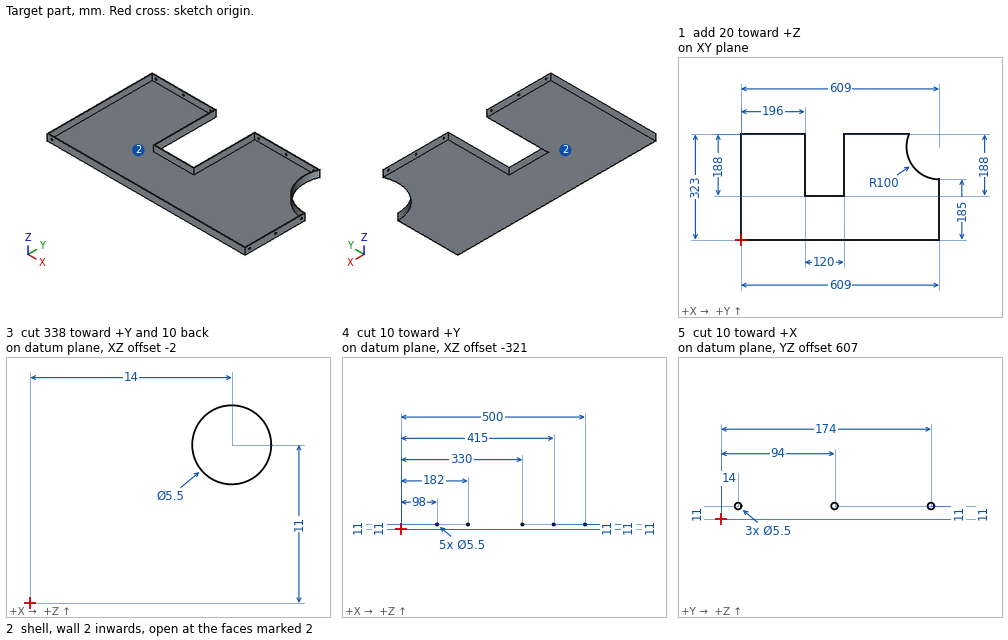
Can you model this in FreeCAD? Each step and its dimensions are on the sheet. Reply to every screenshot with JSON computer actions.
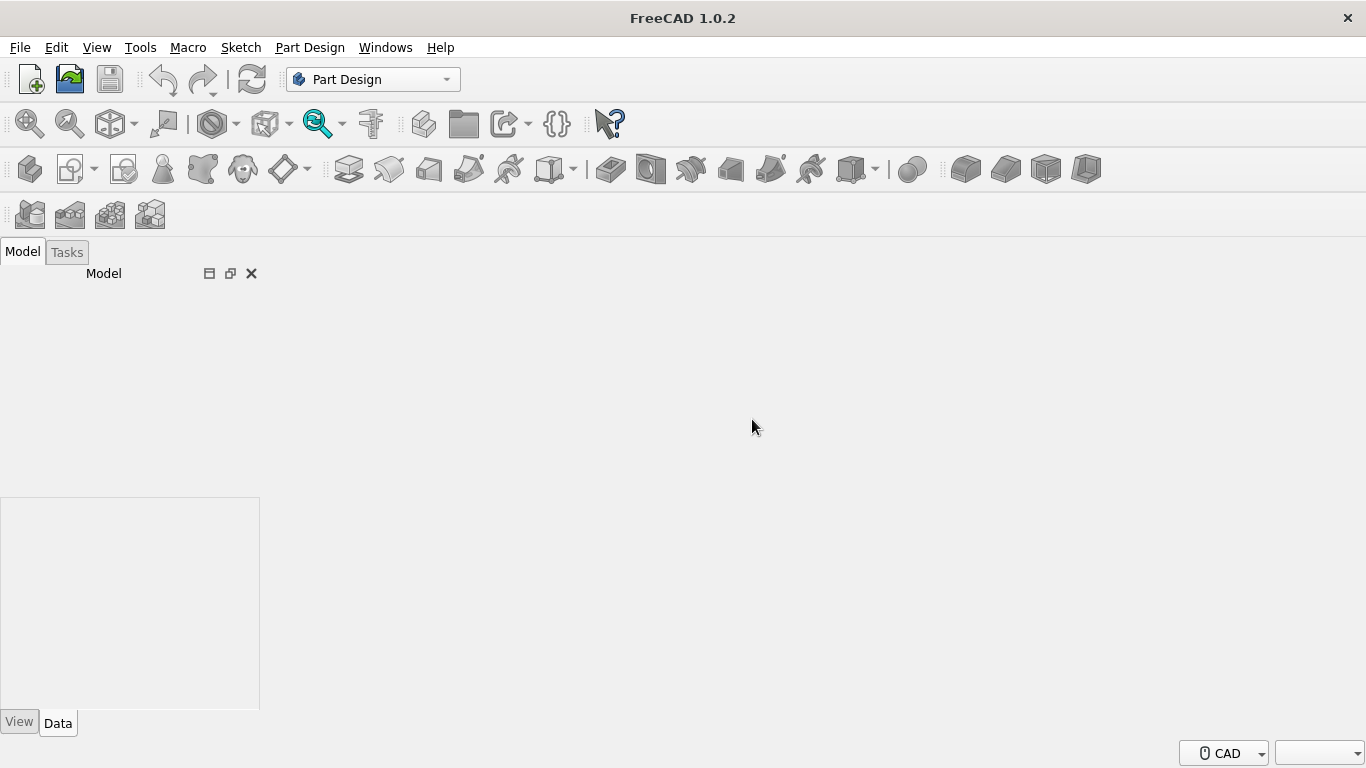
{"action": "key", "text": "ctrl+n"}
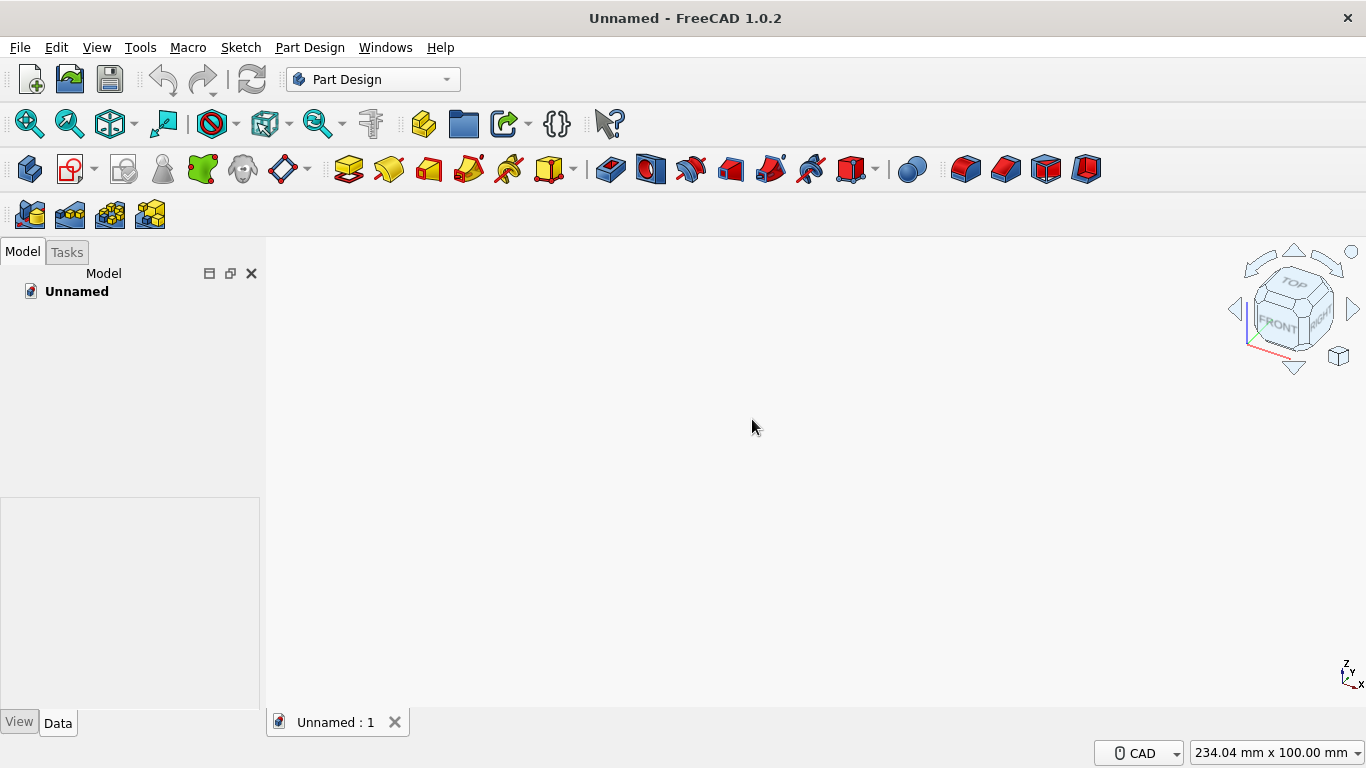
{"action": "left_click", "coordinate": [70, 170]}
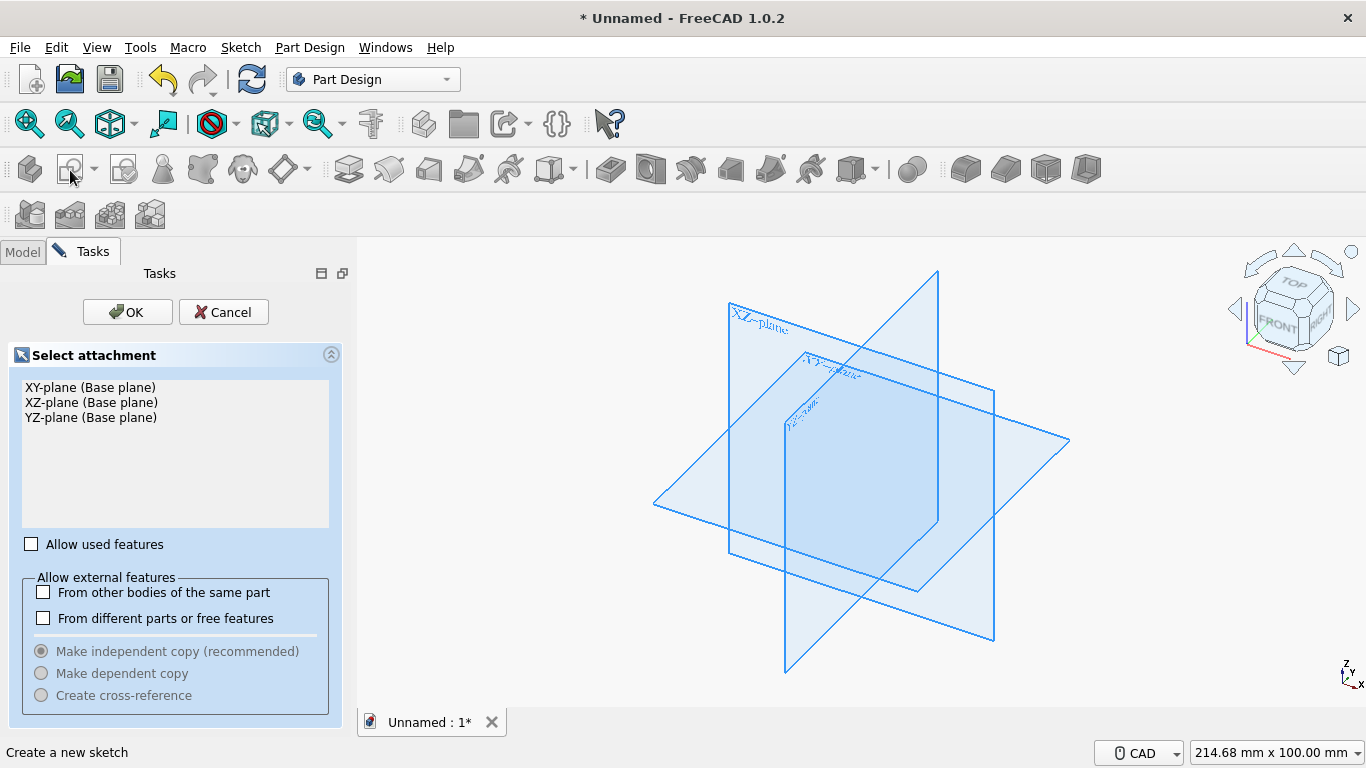
{"action": "left_click", "coordinate": [82, 388]}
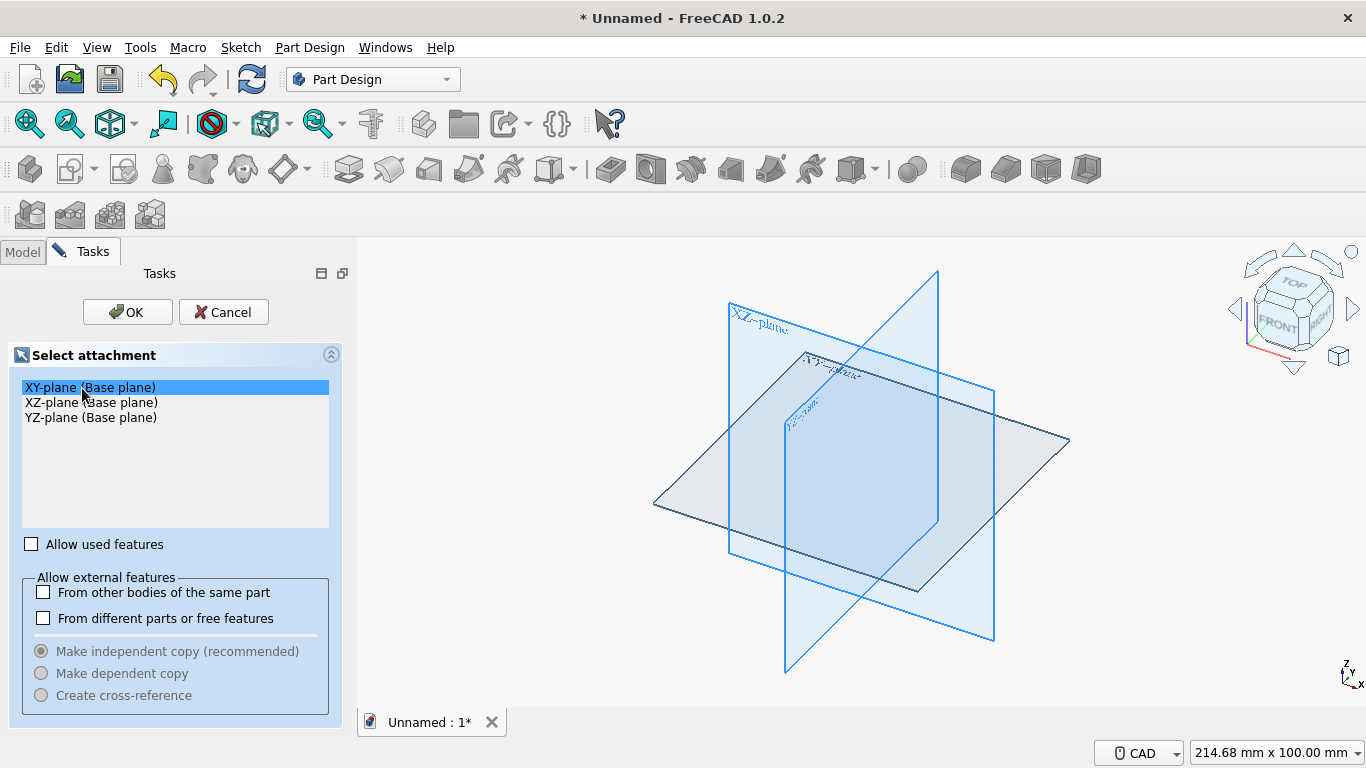
{"action": "left_click", "coordinate": [128, 312]}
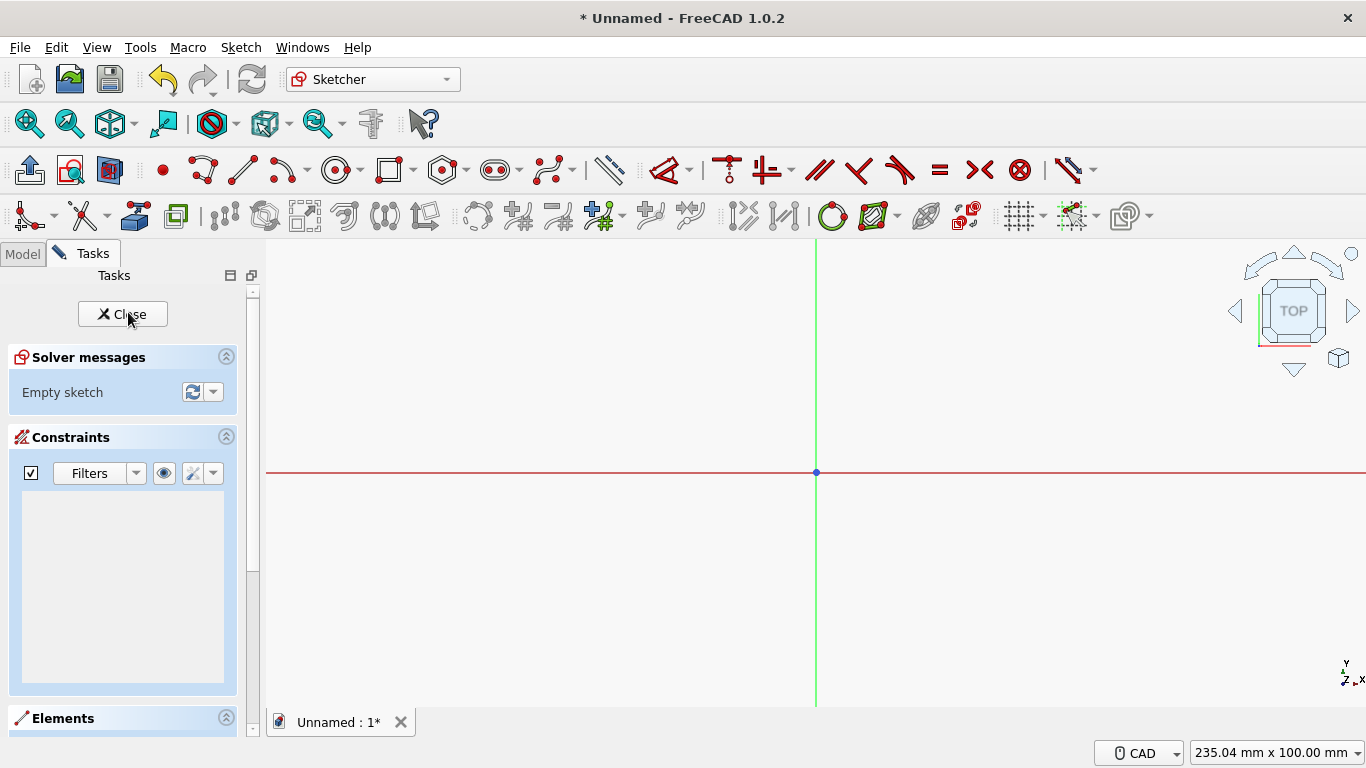
{"action": "scroll", "coordinate": [370, 664], "scroll_direction": "down", "scroll_amount": 8}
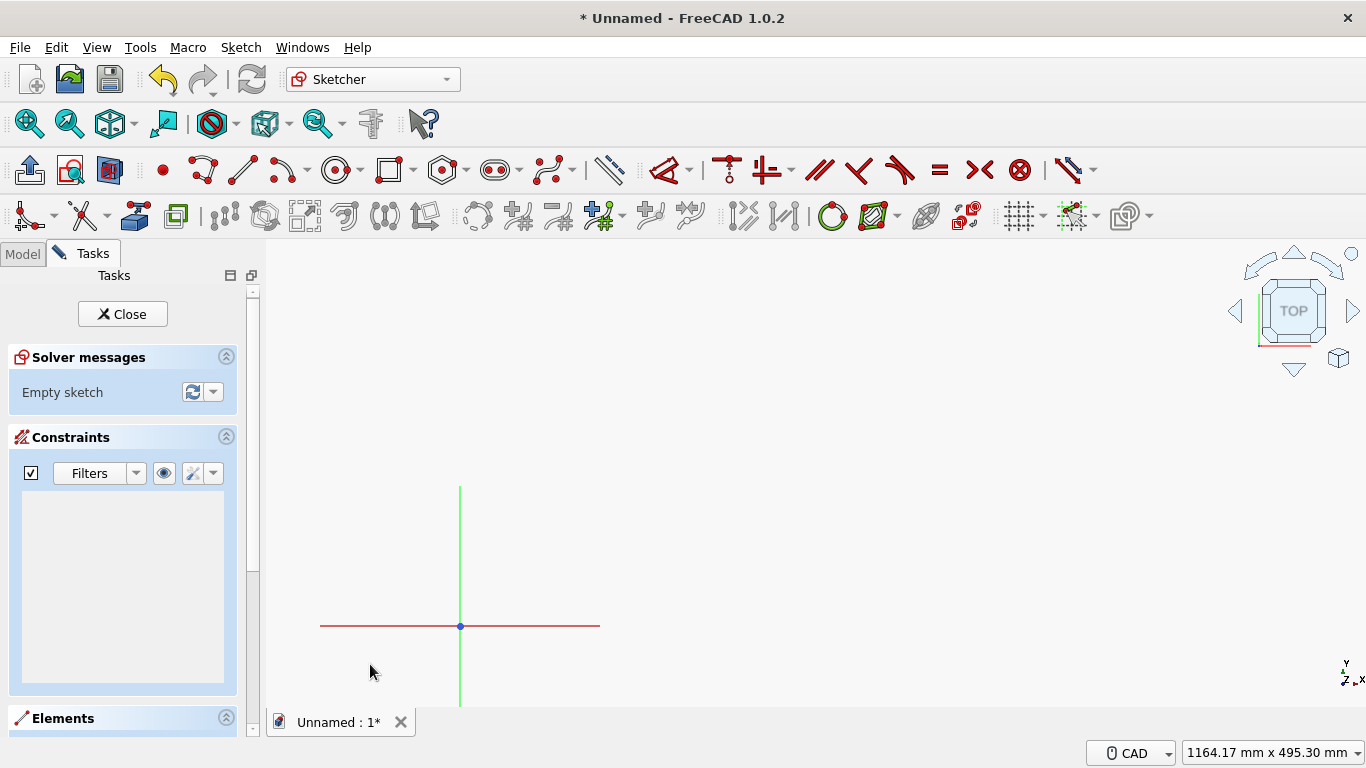
{"action": "key", "text": "g m"}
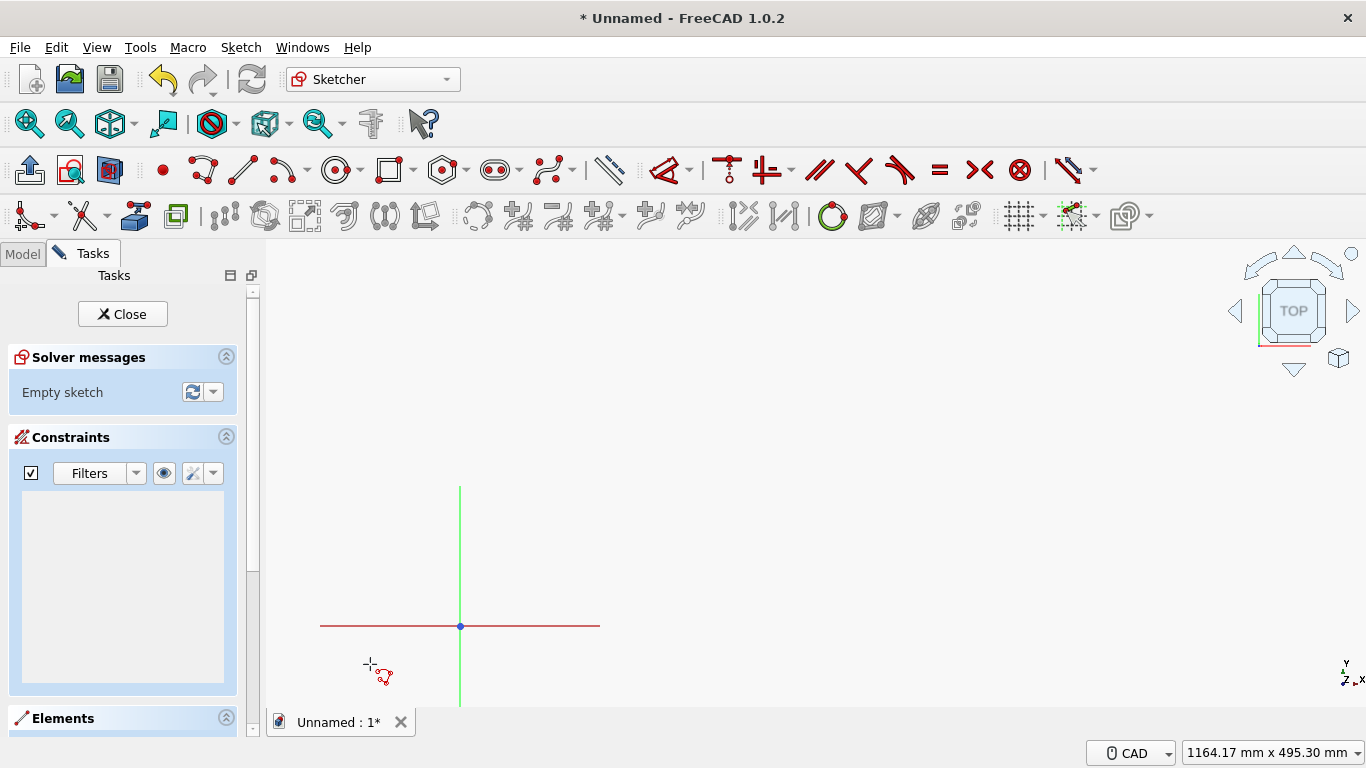
{"action": "left_click", "coordinate": [948, 321]}
{"action": "left_click", "coordinate": [759, 321]}
{"action": "left_click", "coordinate": [759, 499]}
{"action": "left_click", "coordinate": [645, 499]}
{"action": "left_click", "coordinate": [645, 321]}
{"action": "left_click", "coordinate": [460, 321]}
{"action": "left_click", "coordinate": [460, 626]}
{"action": "left_click", "coordinate": [1036, 617]}
{"action": "left_click", "coordinate": [1036, 451]}
{"action": "right_click", "coordinate": [1036, 451]}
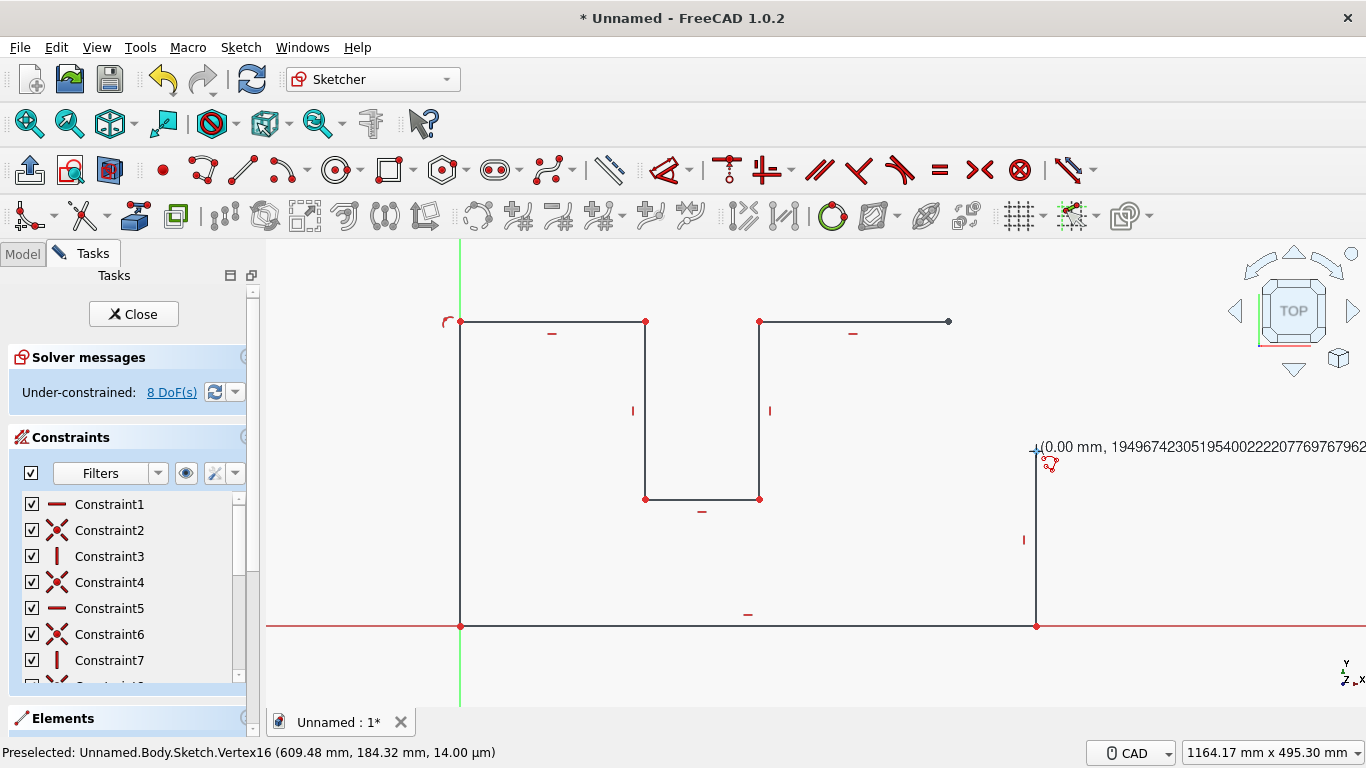
{"action": "left_click", "coordinate": [310, 170]}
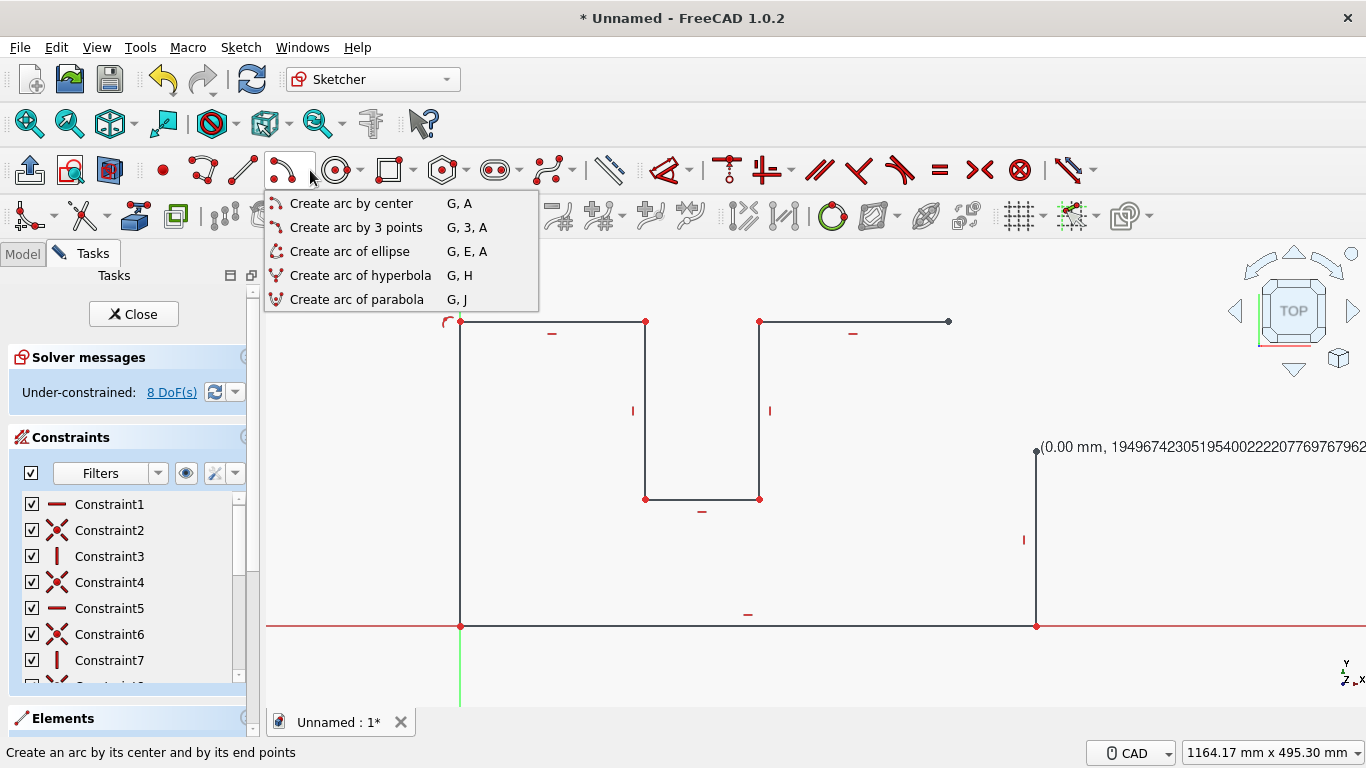
{"action": "left_click", "coordinate": [402, 227]}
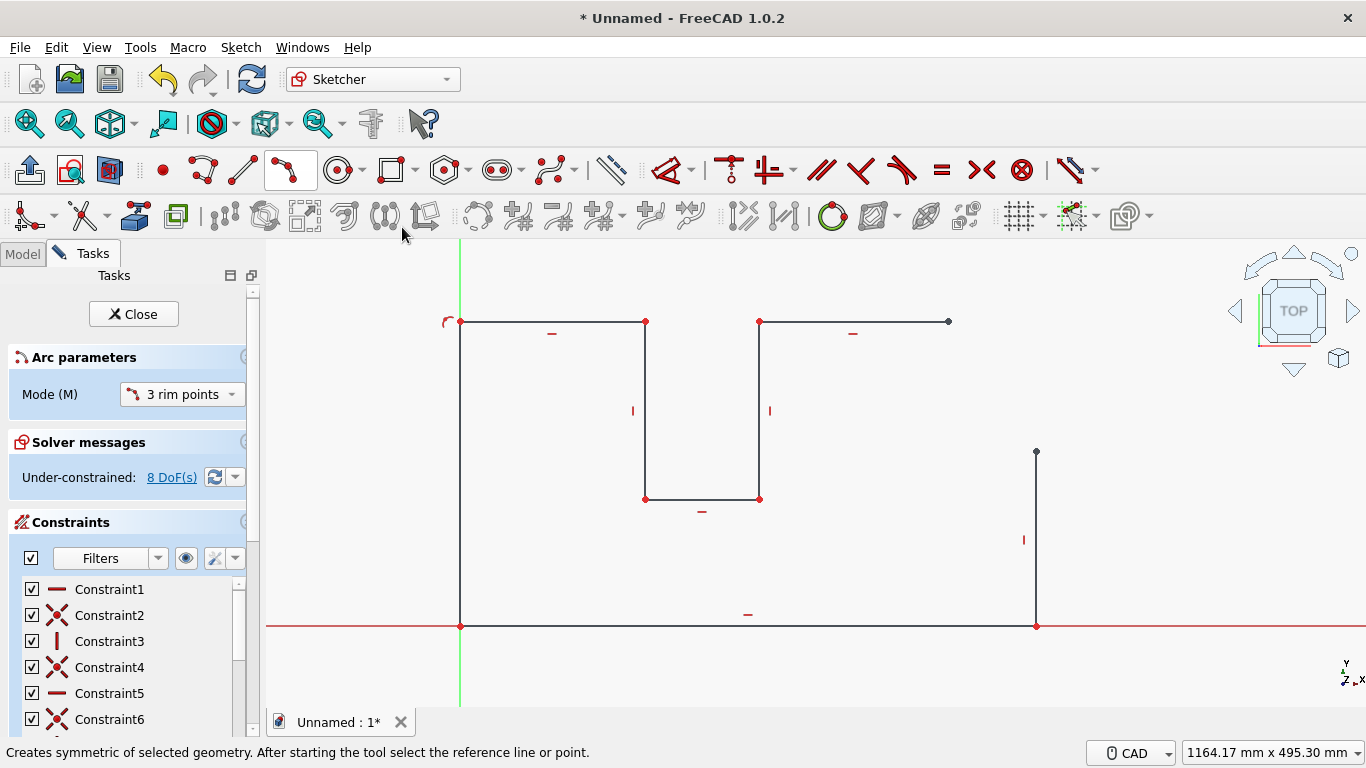
{"action": "left_click", "coordinate": [1036, 452]}
{"action": "left_click", "coordinate": [948, 322]}
{"action": "left_click", "coordinate": [957, 409]}
{"action": "key", "text": "Escape"}